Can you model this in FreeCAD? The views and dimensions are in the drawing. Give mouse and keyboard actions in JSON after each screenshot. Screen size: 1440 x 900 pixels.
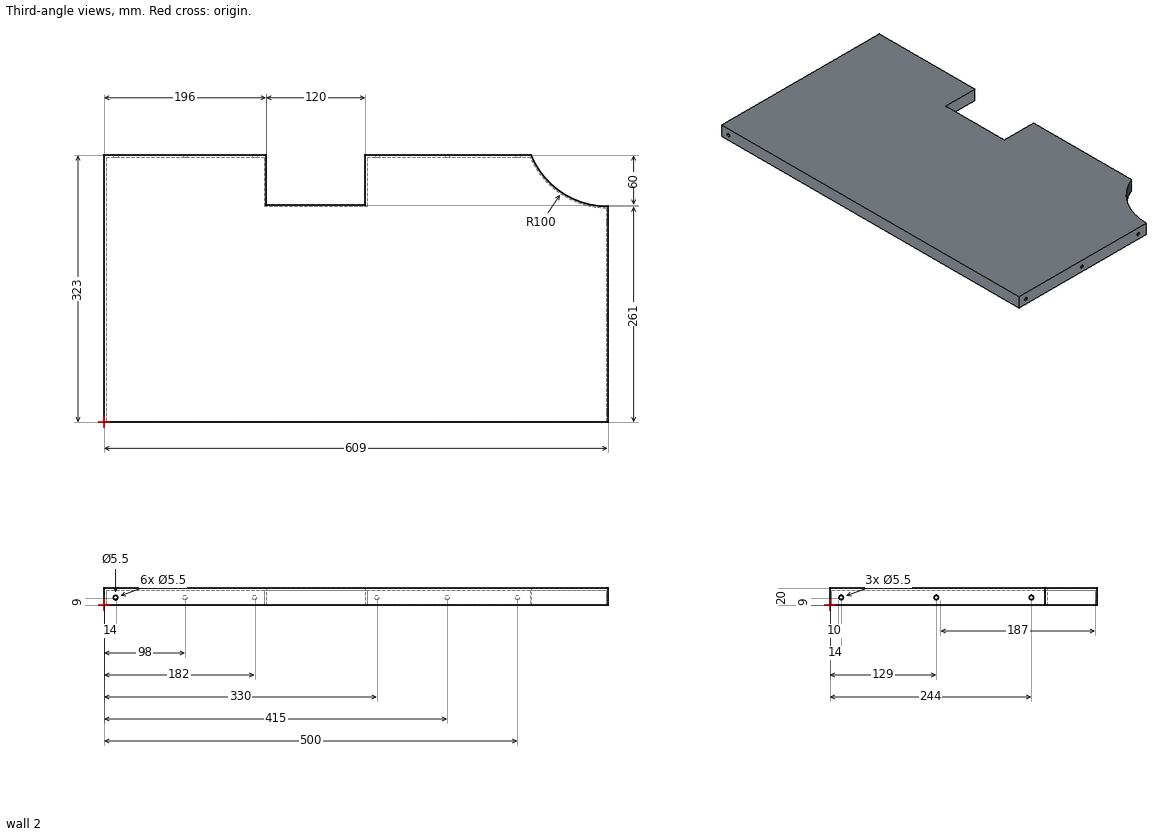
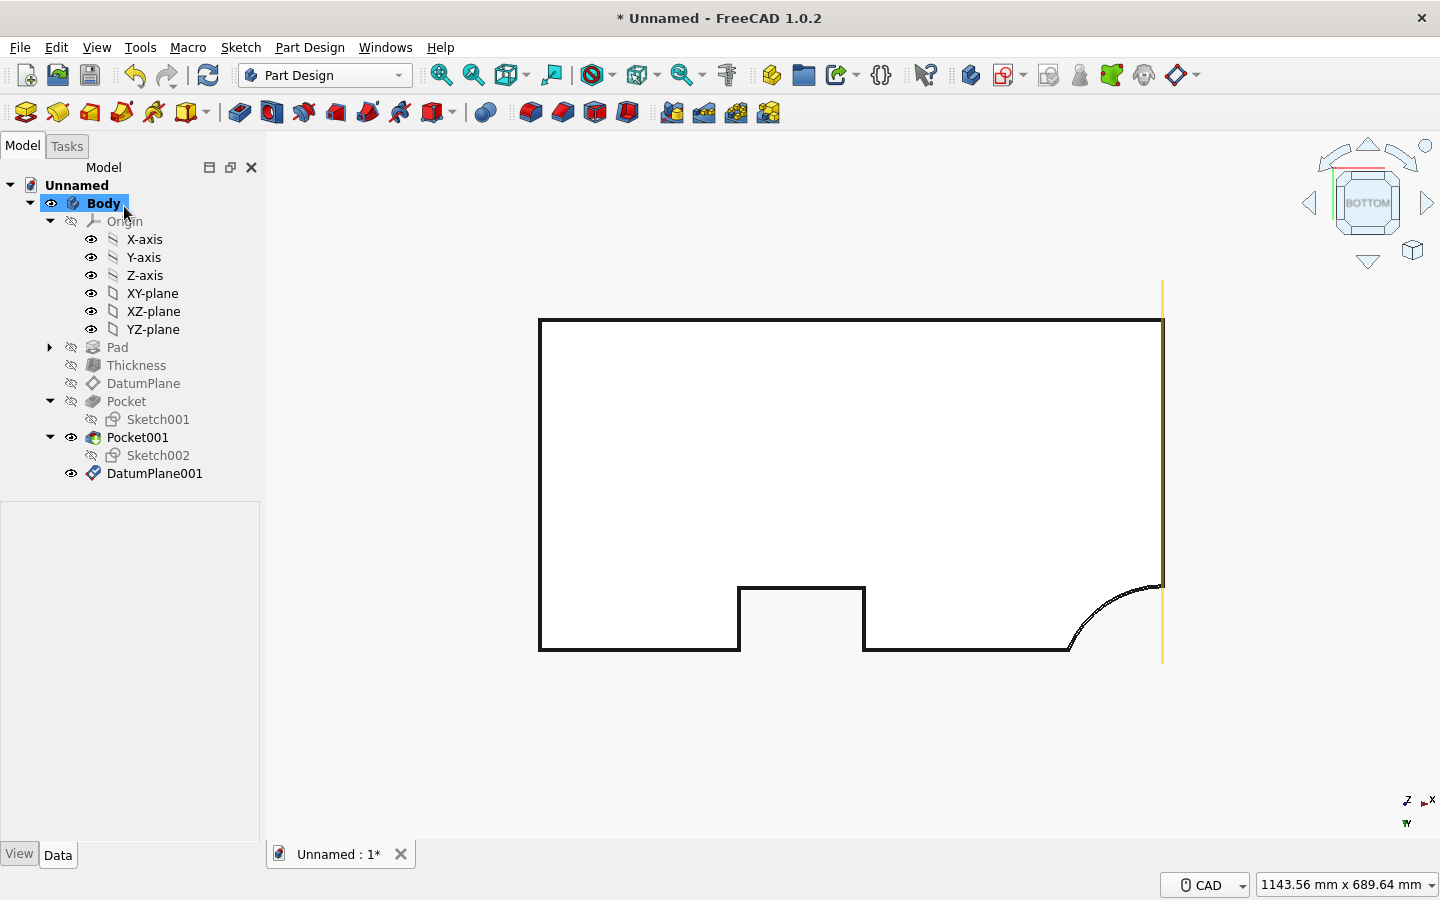
{"action": "left_click", "coordinate": [116, 473]}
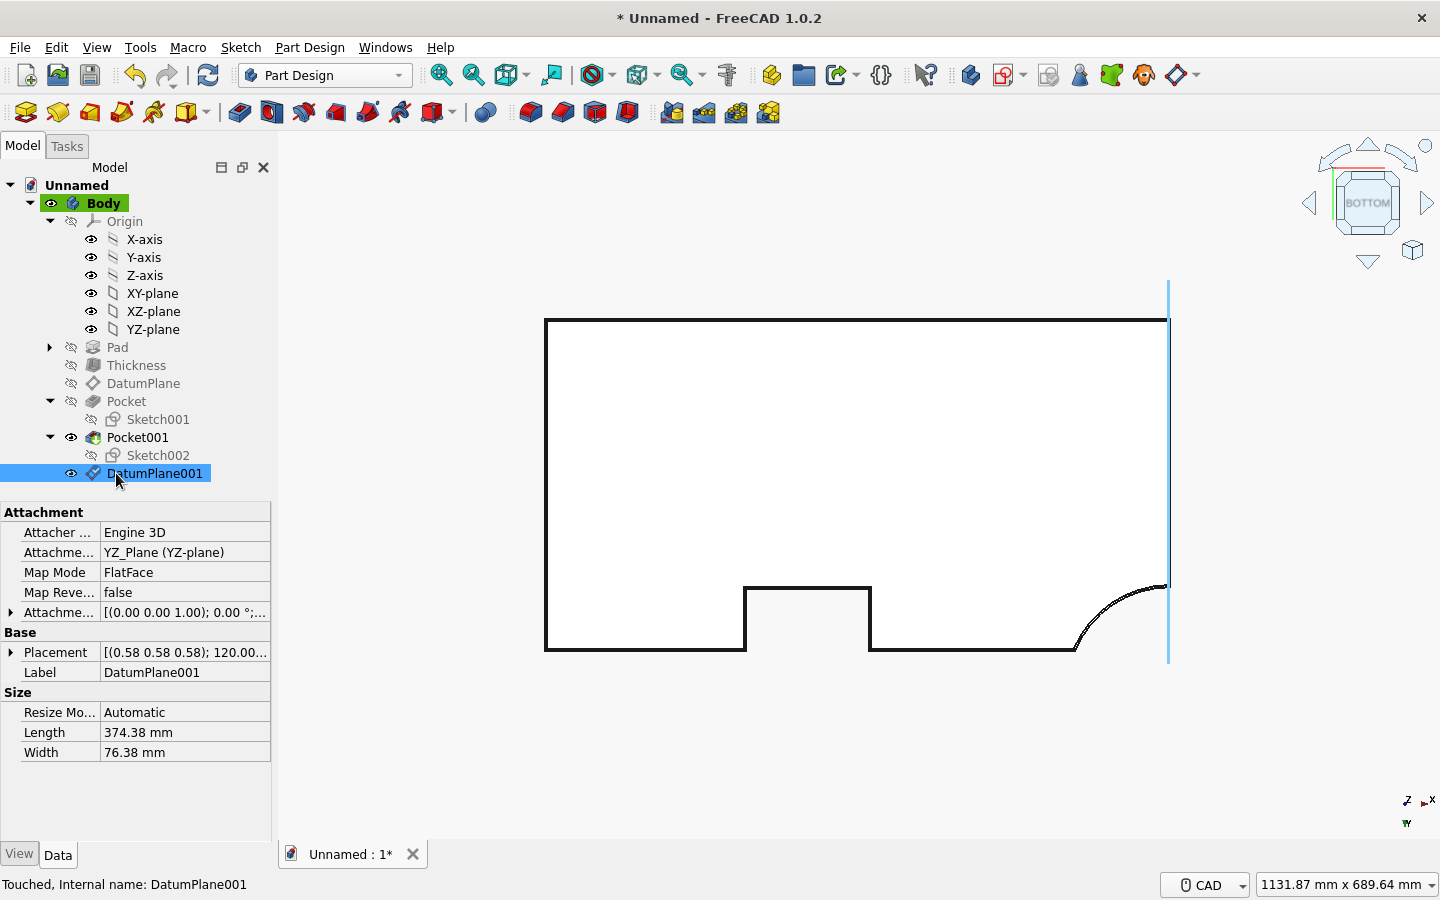
{"action": "left_click", "coordinate": [1004, 76]}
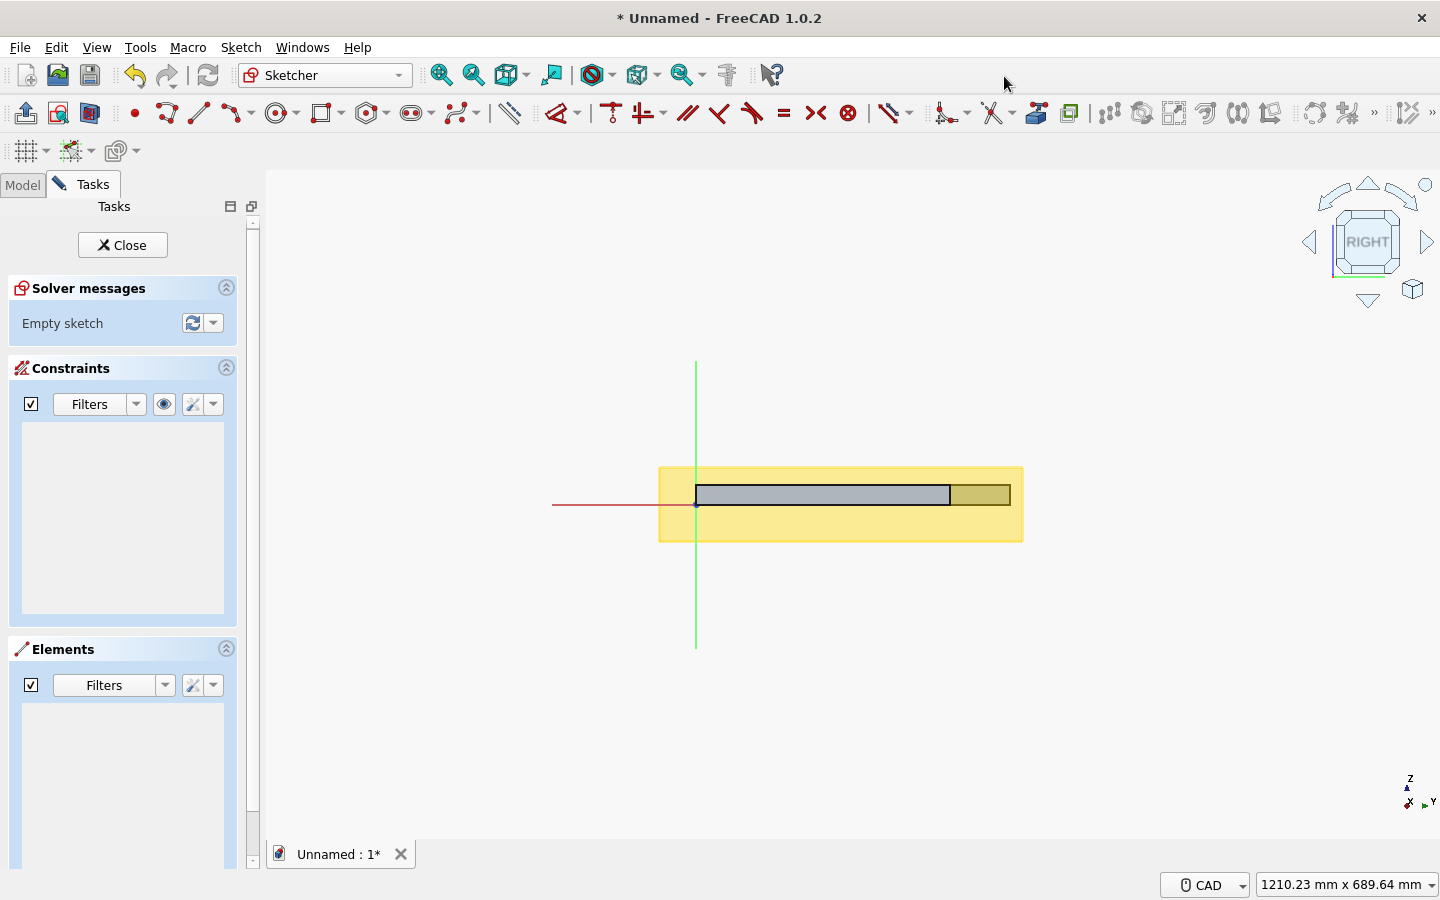
{"action": "key", "text": "q s"}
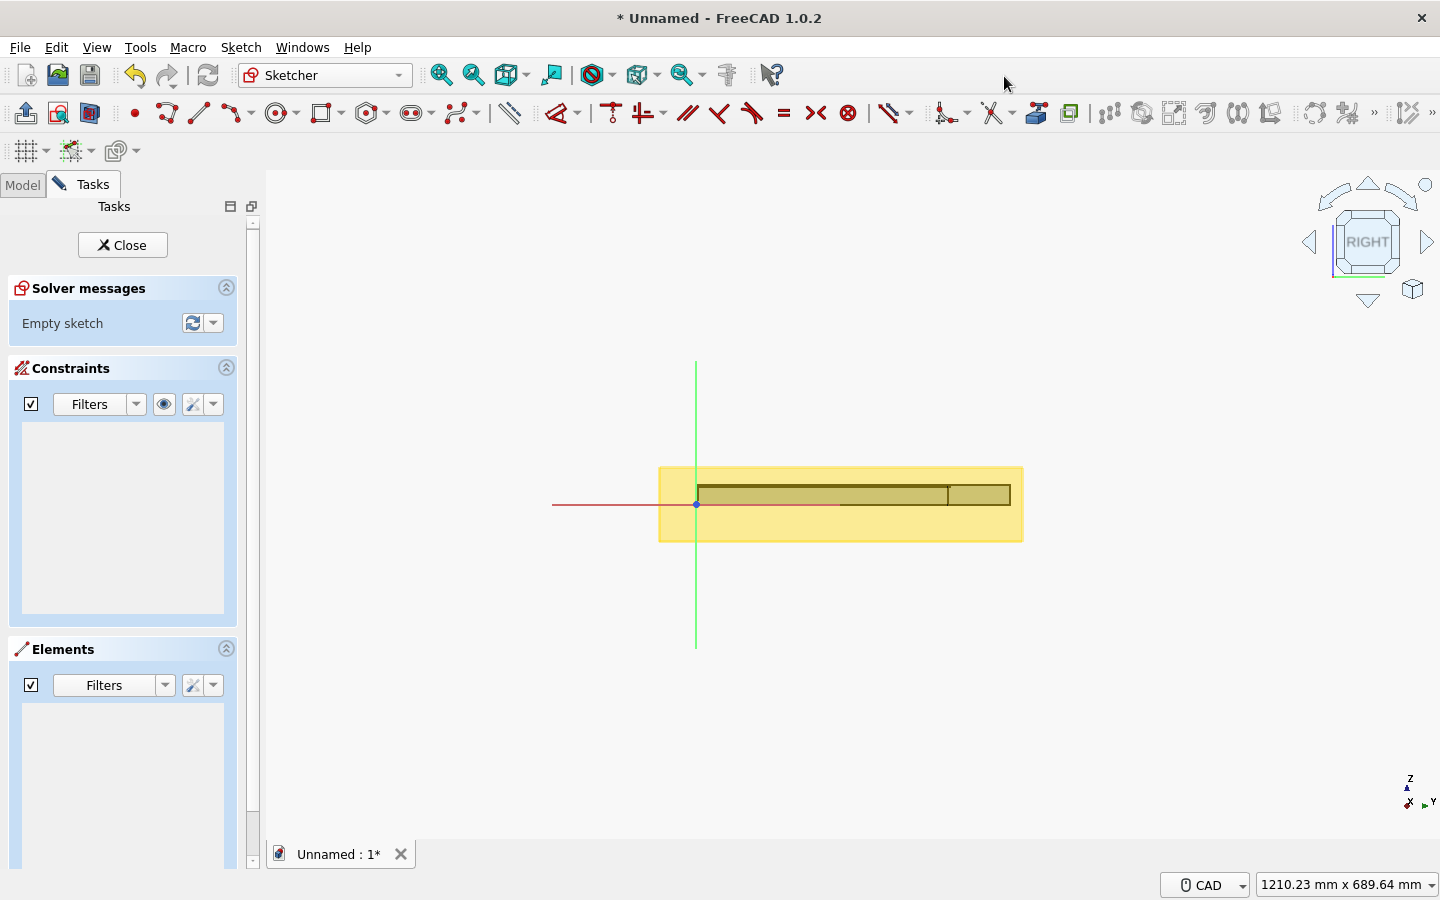
{"action": "scroll", "coordinate": [834, 496], "scroll_direction": "up", "scroll_amount": 5}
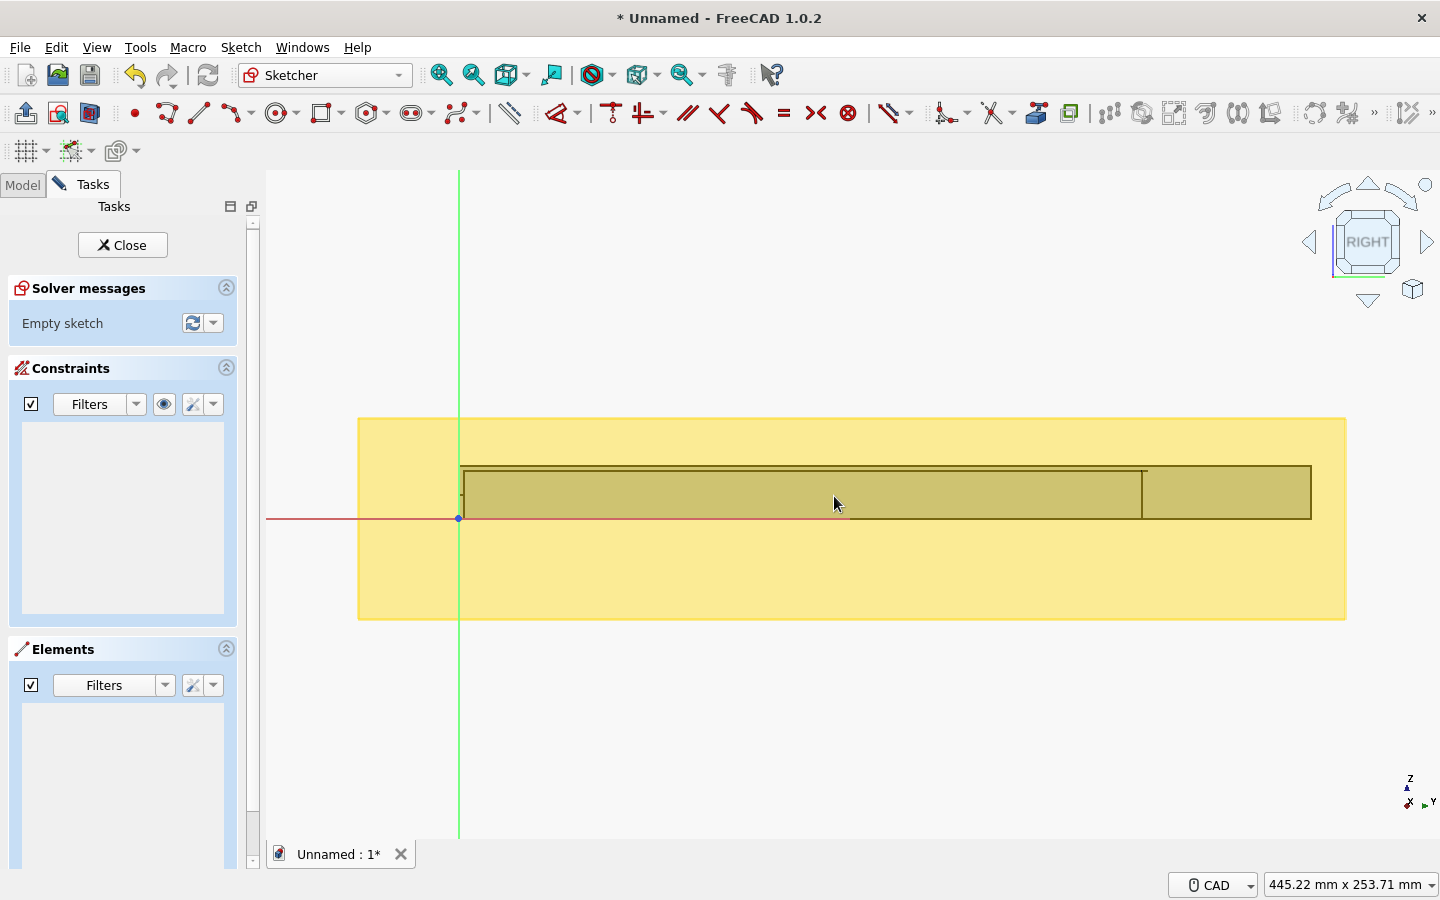
{"action": "key", "text": "g c"}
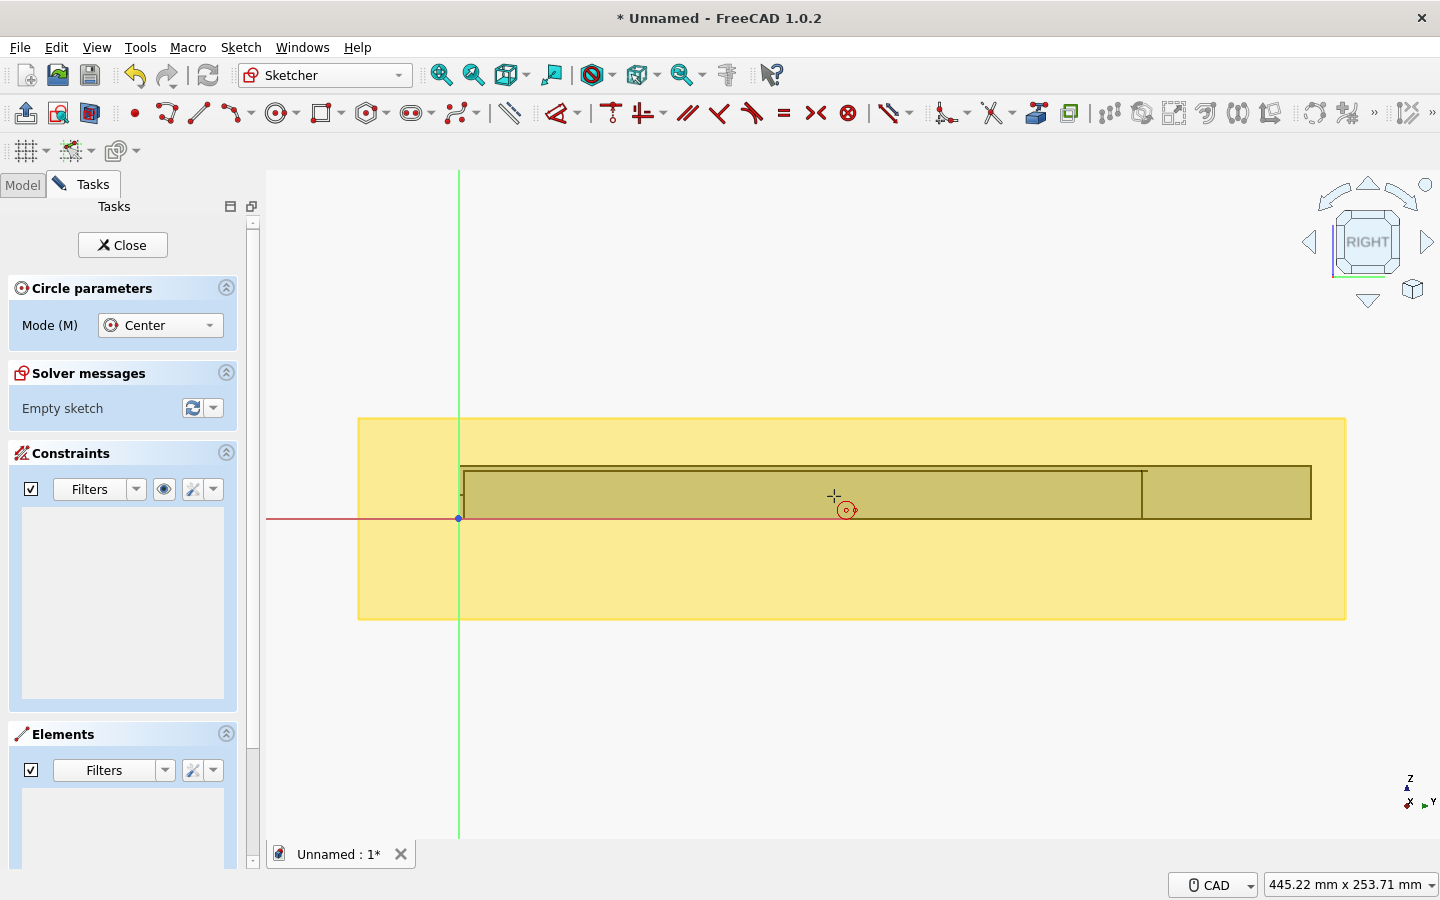
{"action": "scroll", "coordinate": [496, 495], "scroll_direction": "up", "scroll_amount": 6}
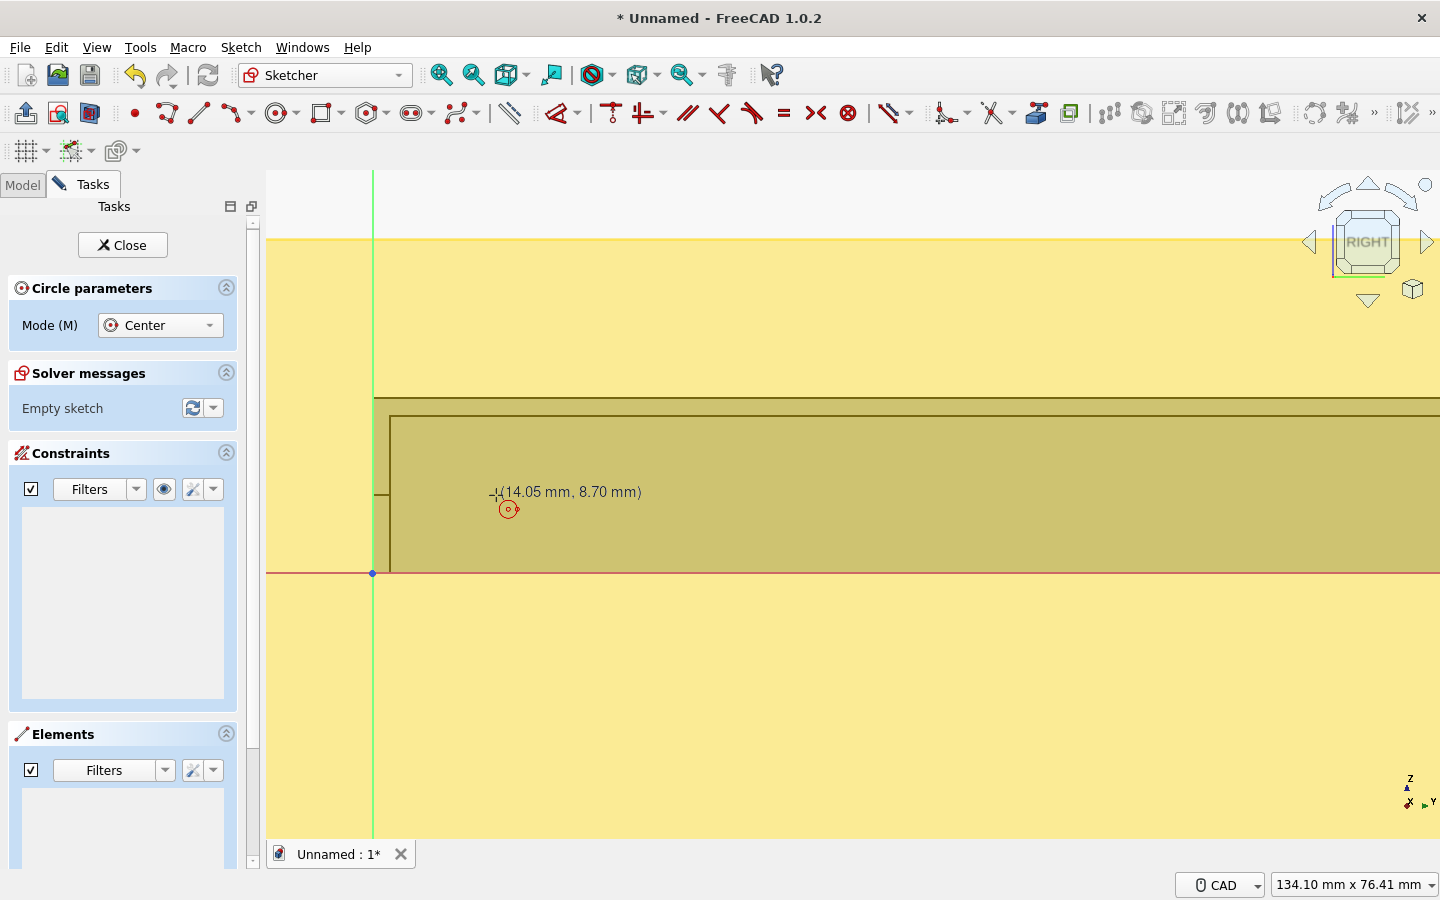
{"action": "left_click", "coordinate": [495, 495]}
{"action": "mouse_move", "coordinate": [512, 478]}